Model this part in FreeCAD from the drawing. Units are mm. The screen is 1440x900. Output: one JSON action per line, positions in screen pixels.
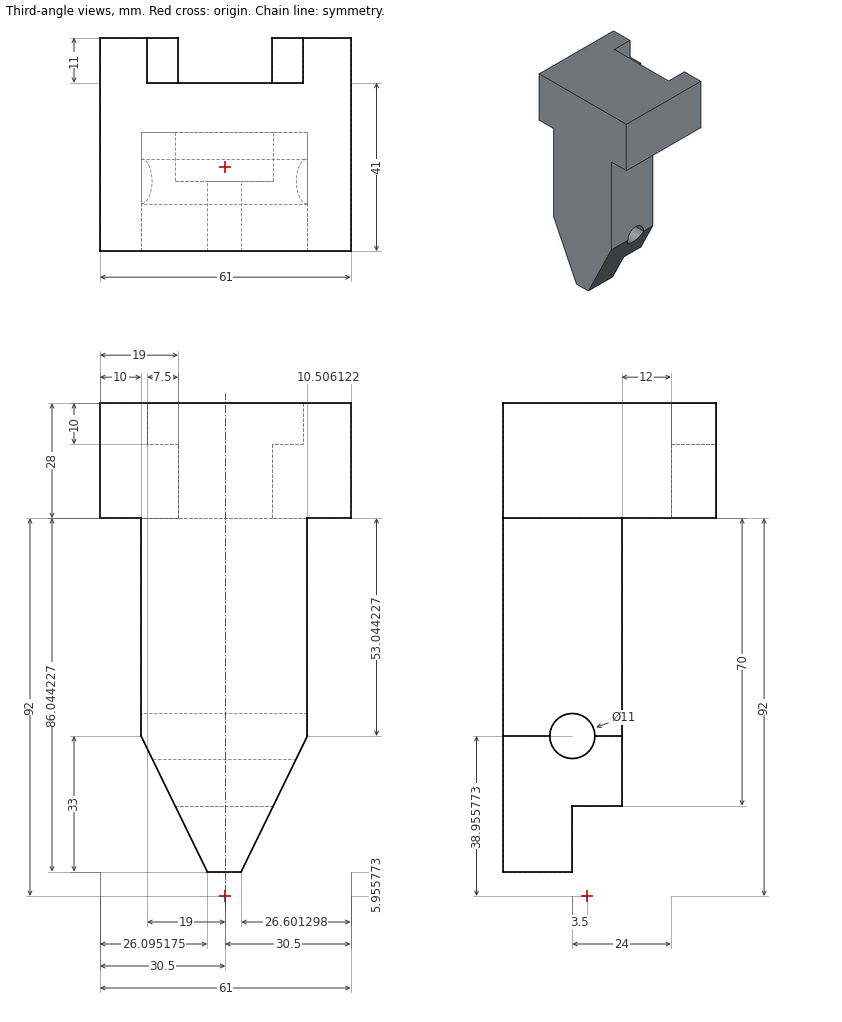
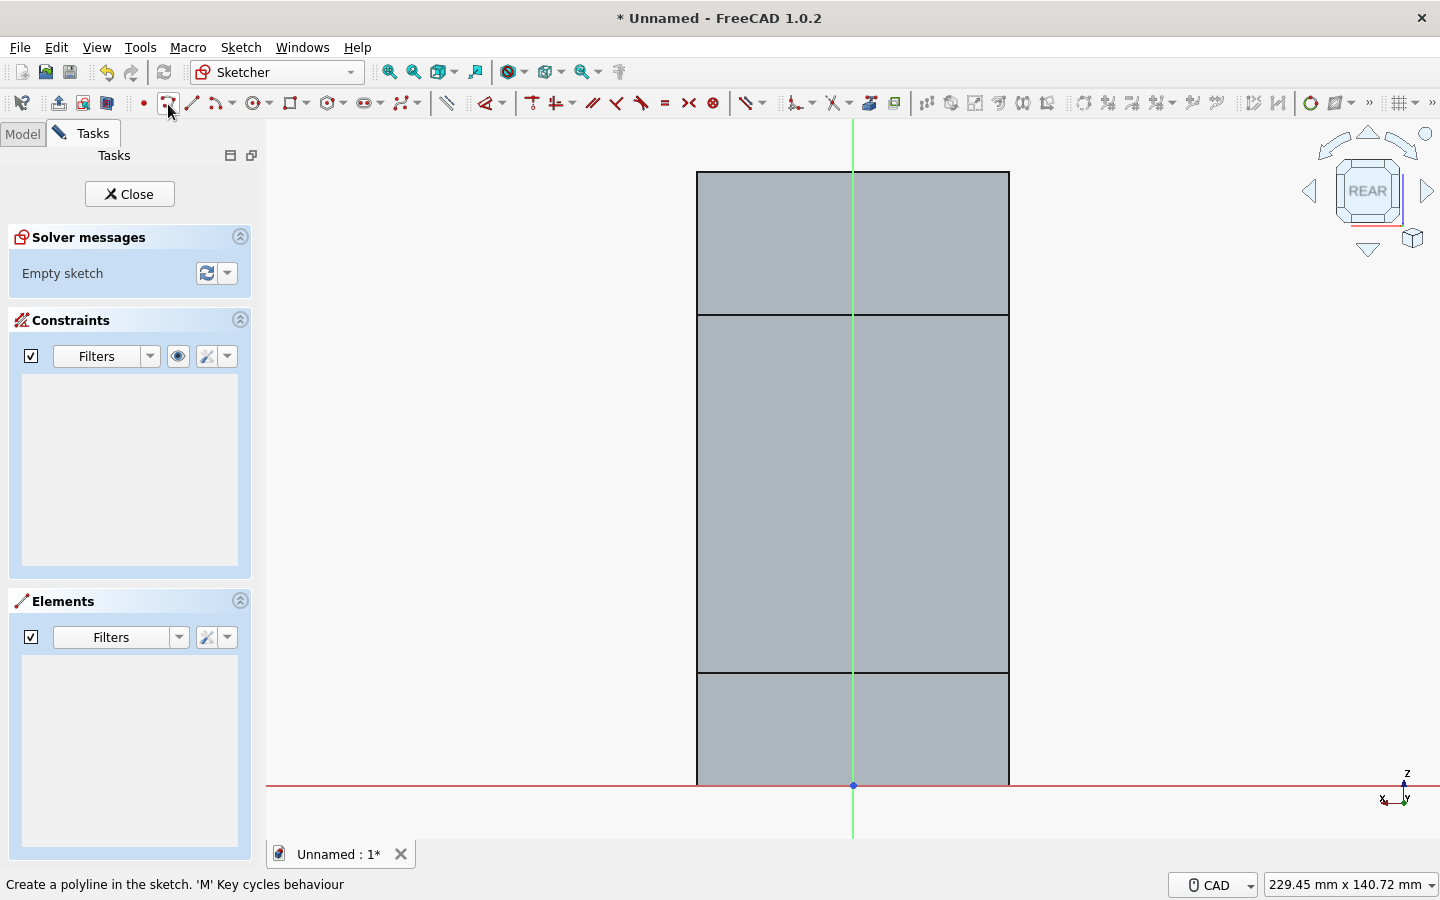
{"action": "left_click", "coordinate": [912, 315]}
{"action": "left_click", "coordinate": [1009, 315]}
{"action": "left_click", "coordinate": [1009, 172]}
{"action": "left_click", "coordinate": [950, 172]}
{"action": "left_click", "coordinate": [950, 223]}
{"action": "left_click", "coordinate": [912, 223]}
{"action": "left_click", "coordinate": [912, 316]}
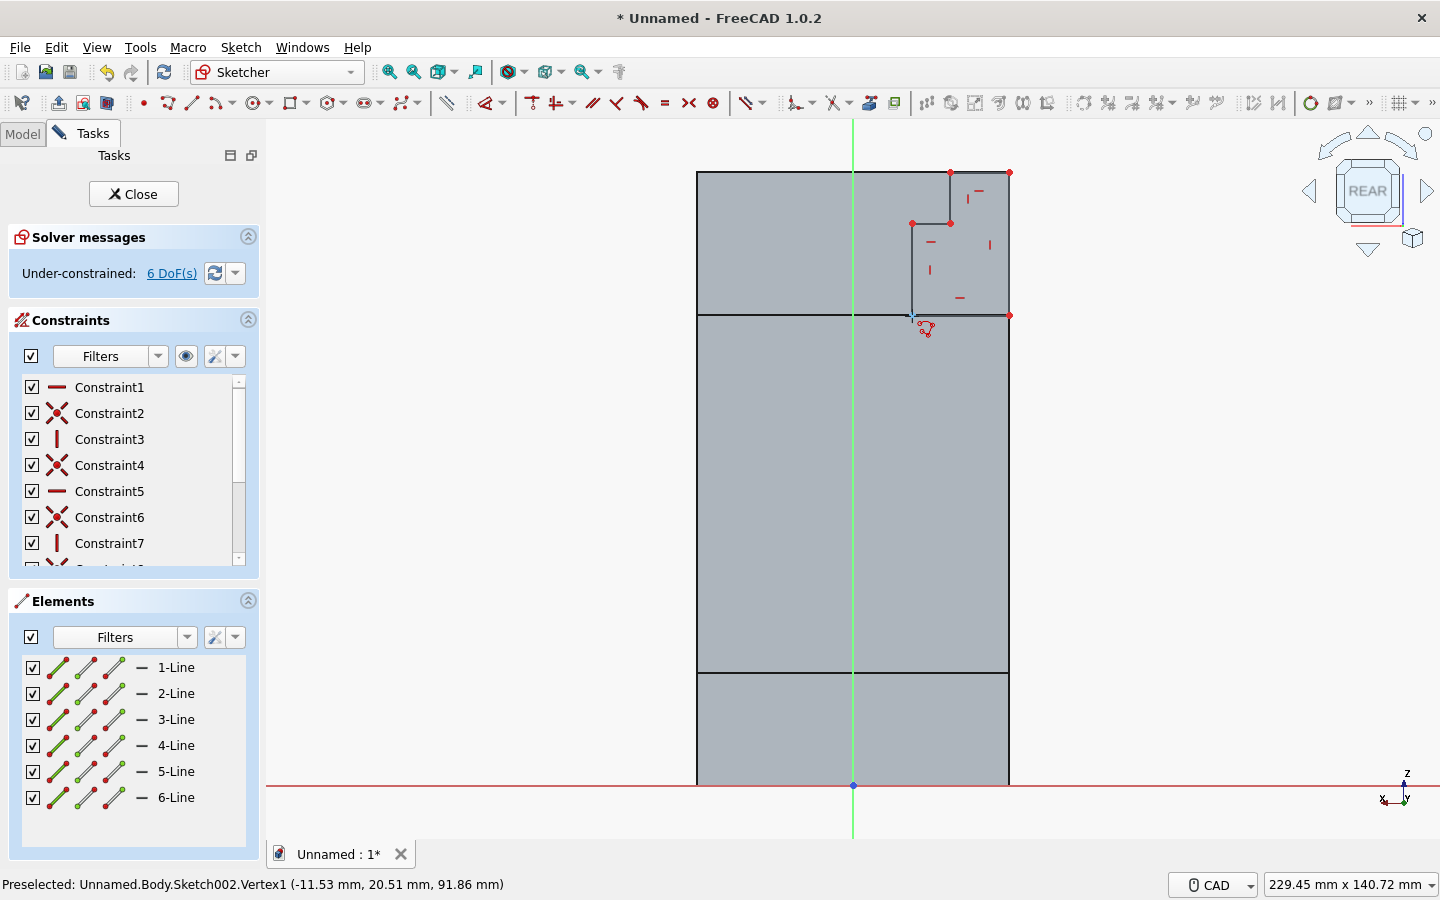
{"action": "left_click", "coordinate": [794, 315]}
{"action": "left_click", "coordinate": [794, 223]}
{"action": "left_click", "coordinate": [756, 223]}
{"action": "left_click", "coordinate": [756, 172]}
{"action": "left_click", "coordinate": [697, 172]}
{"action": "left_click", "coordinate": [697, 315]}
{"action": "left_click", "coordinate": [794, 316]}
{"action": "key", "text": "Escape"}
{"action": "key", "text": "Escape"}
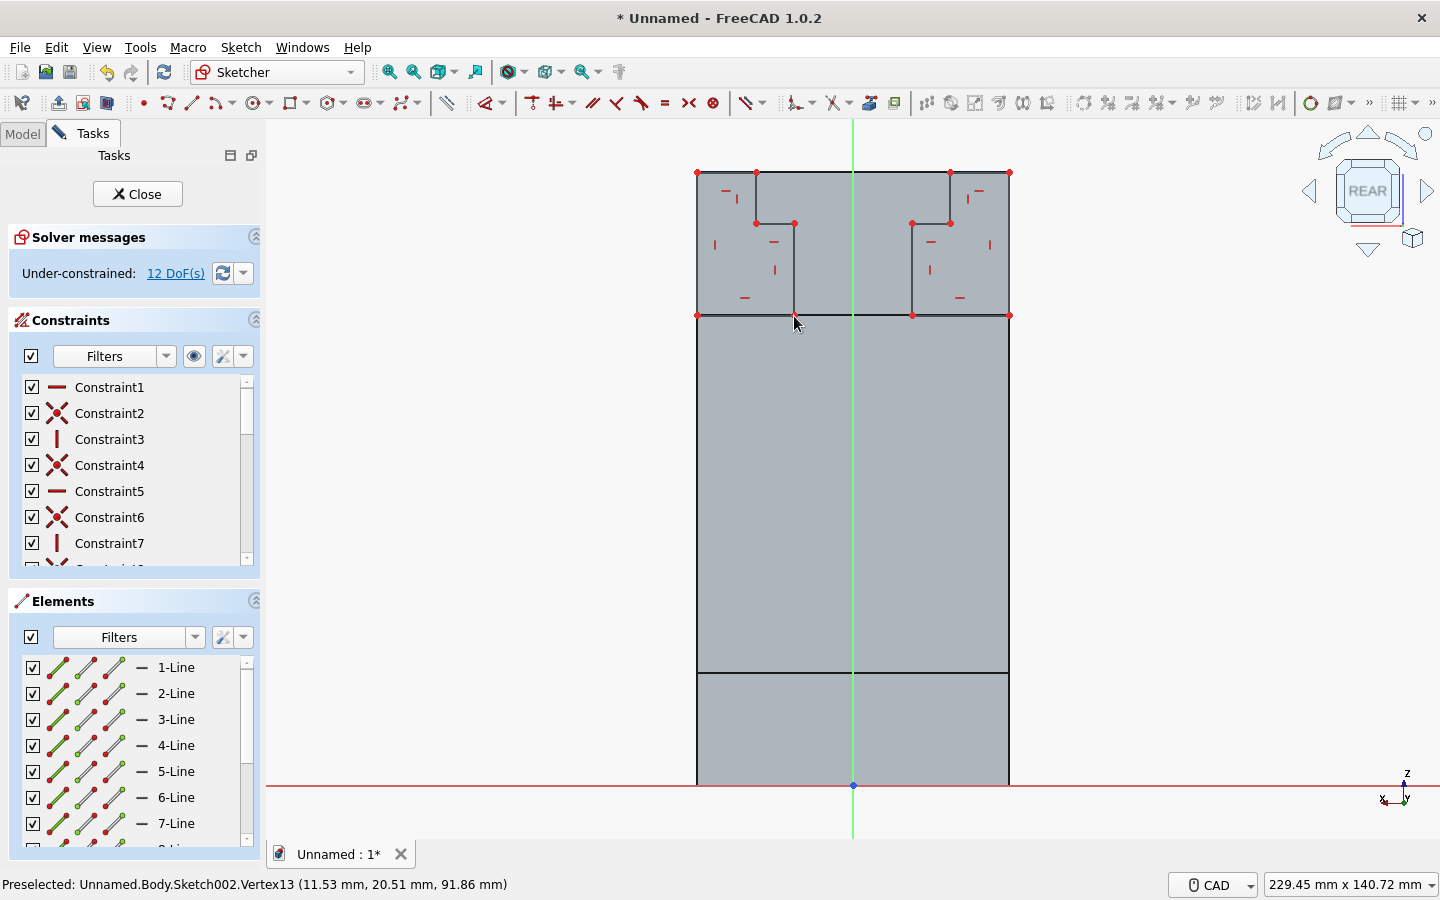
{"action": "left_click", "coordinate": [912, 316]}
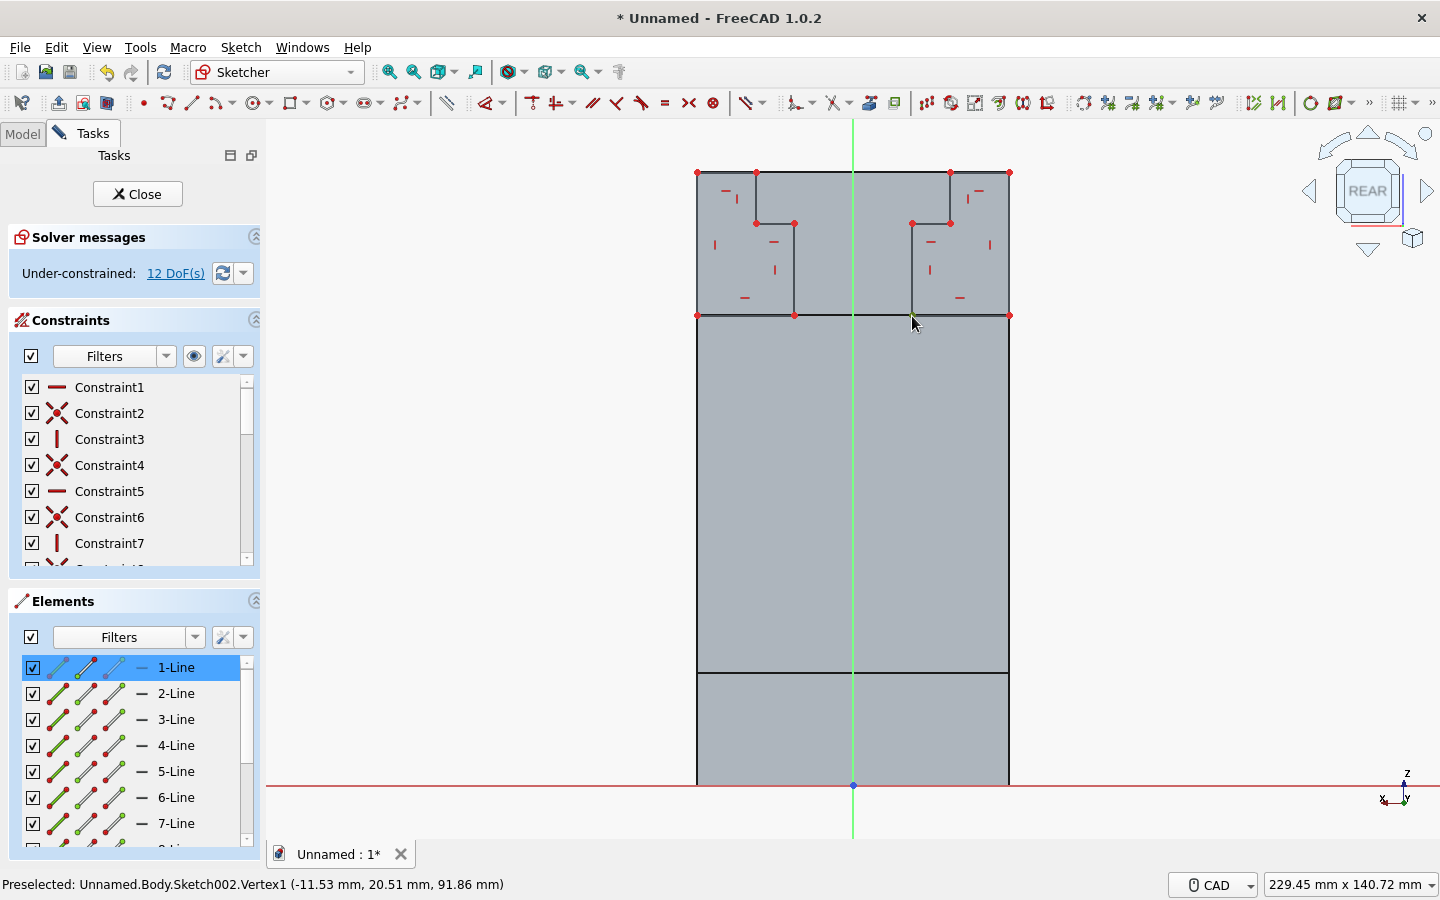
{"action": "left_click", "coordinate": [794, 316]}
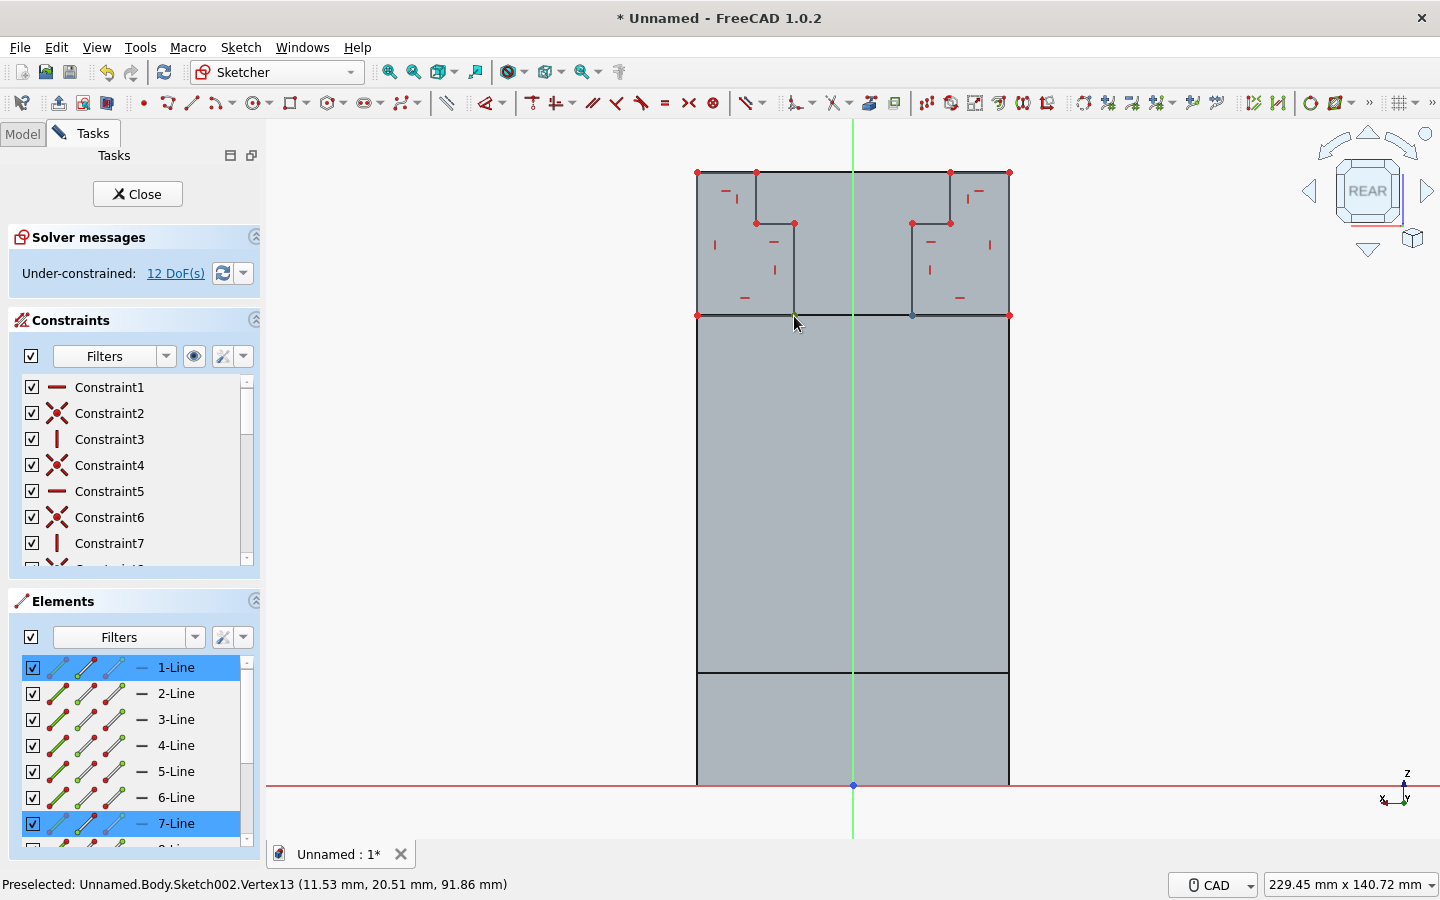
{"action": "left_click", "coordinate": [853, 716]}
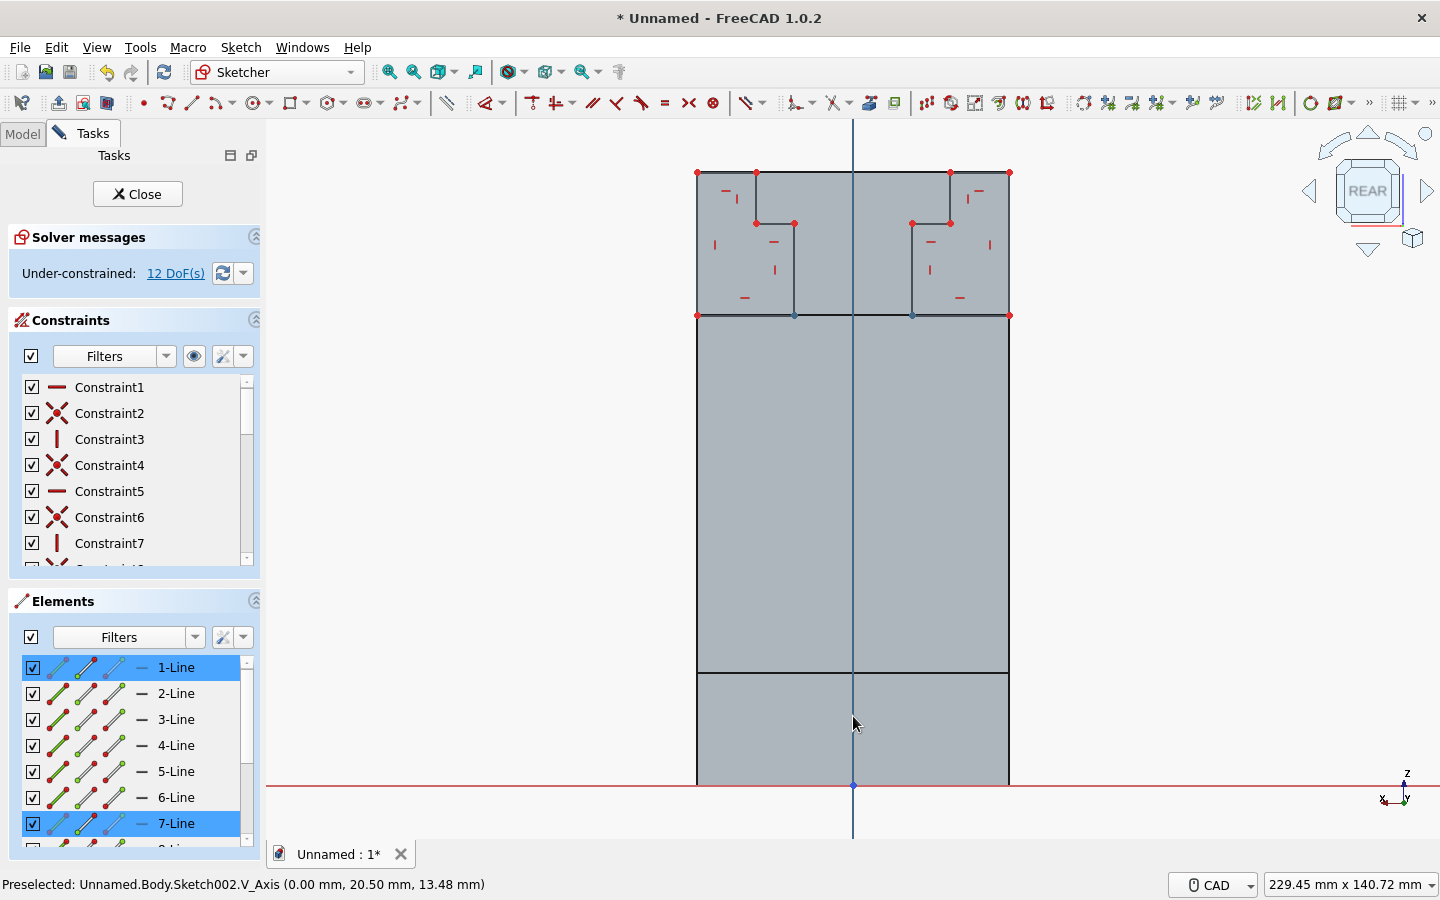
{"action": "left_click", "coordinate": [690, 104]}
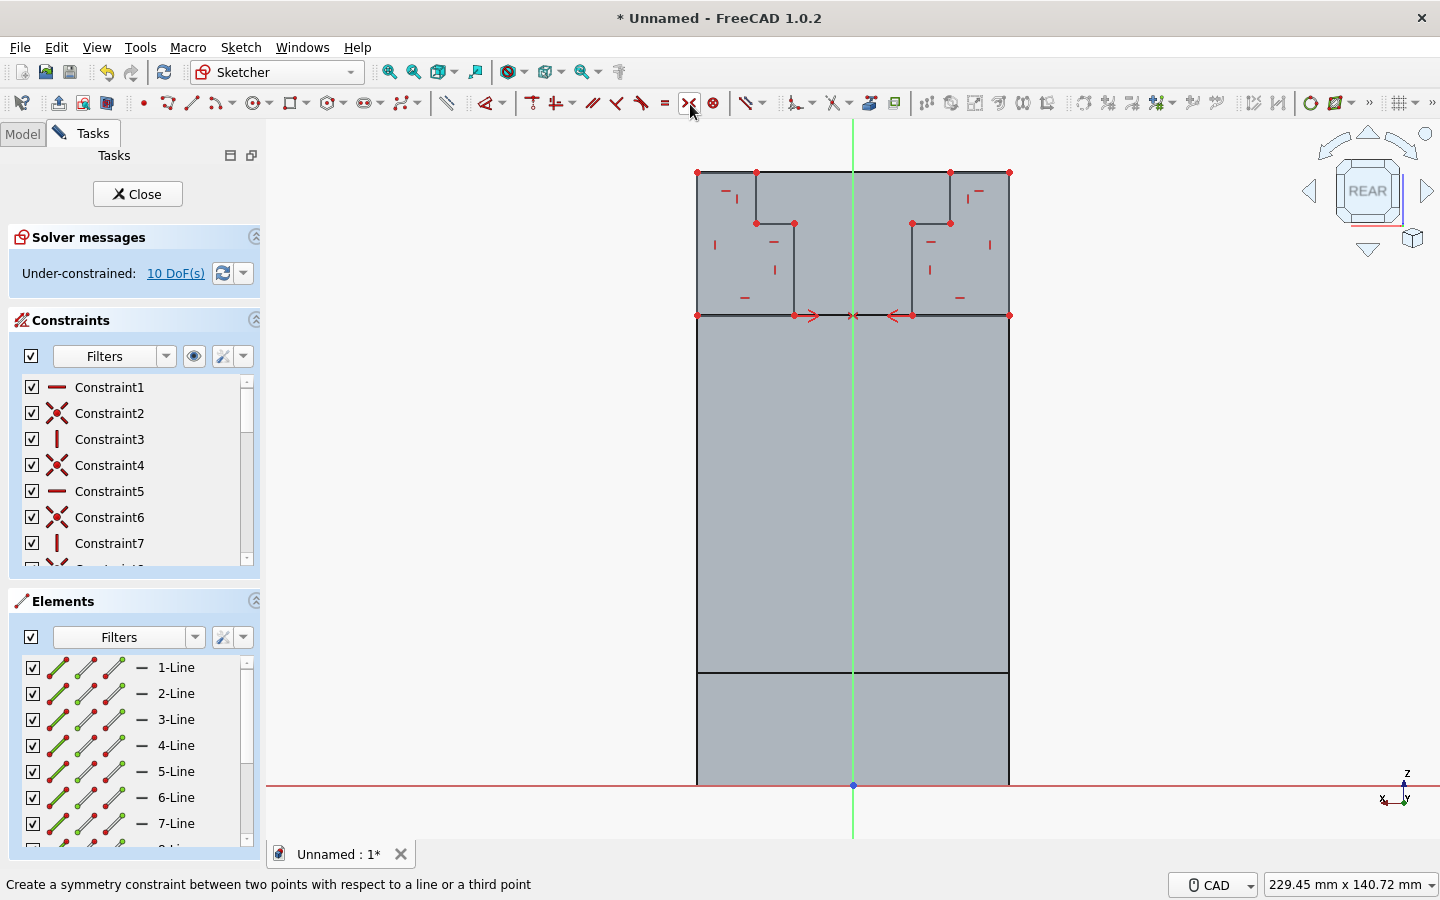
{"action": "left_click", "coordinate": [950, 224]}